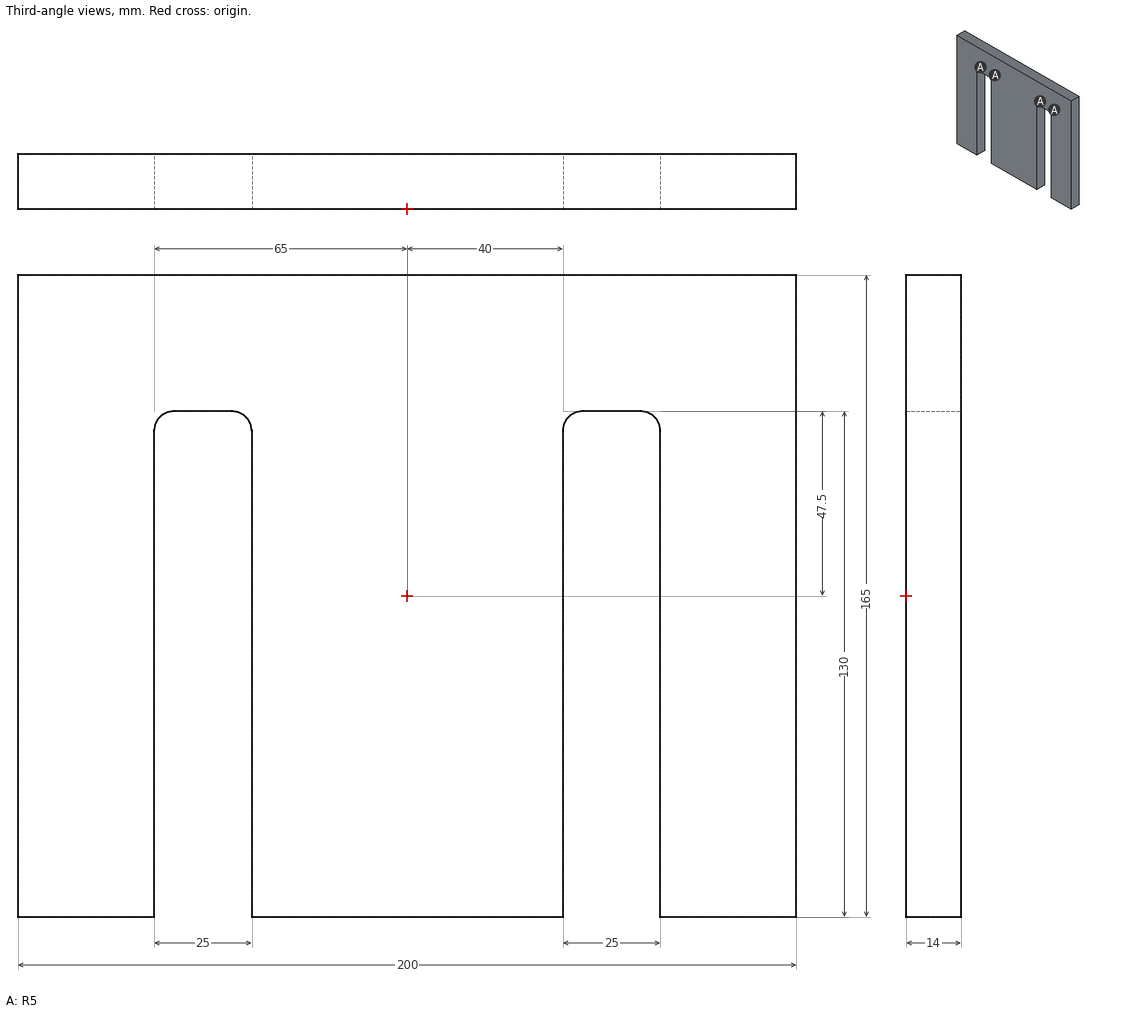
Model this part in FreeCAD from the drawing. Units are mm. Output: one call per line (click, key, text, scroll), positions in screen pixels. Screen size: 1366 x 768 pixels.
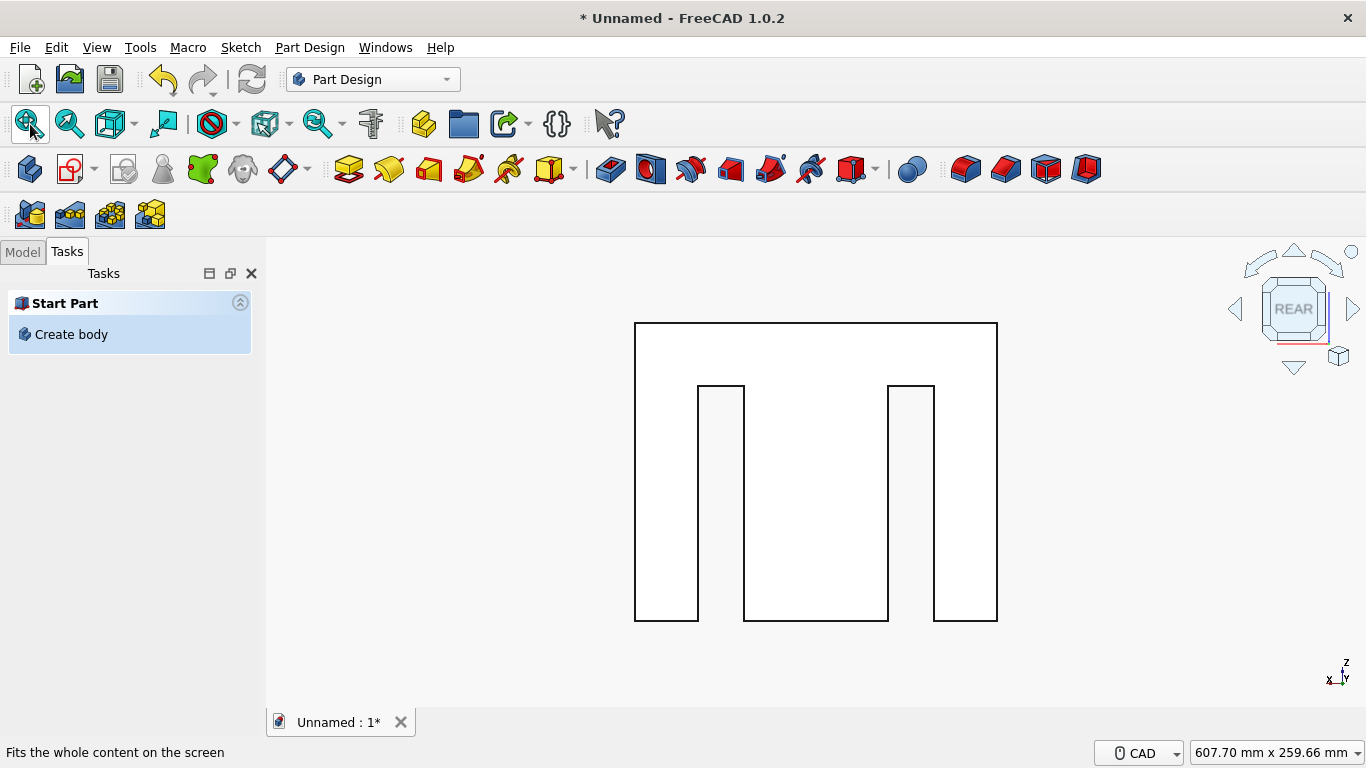
key(6)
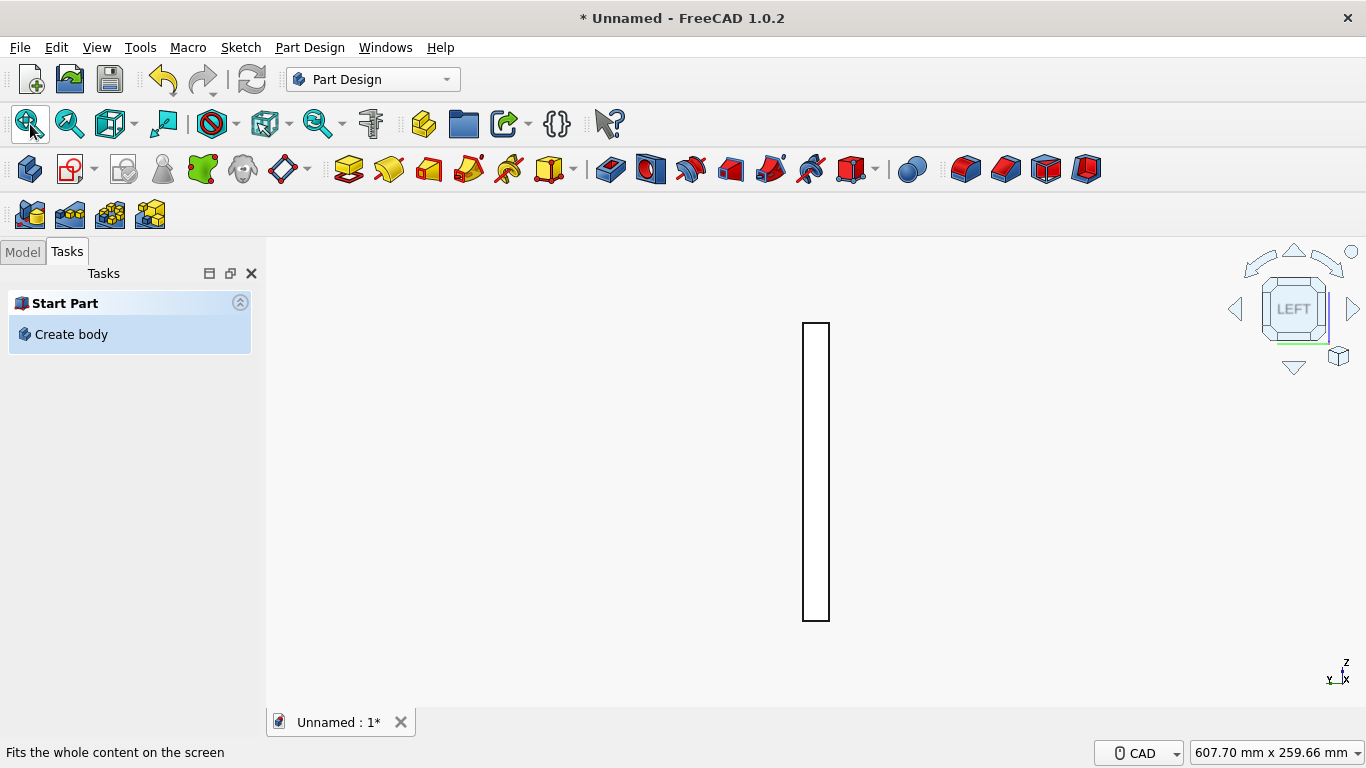
key(v)
key(3)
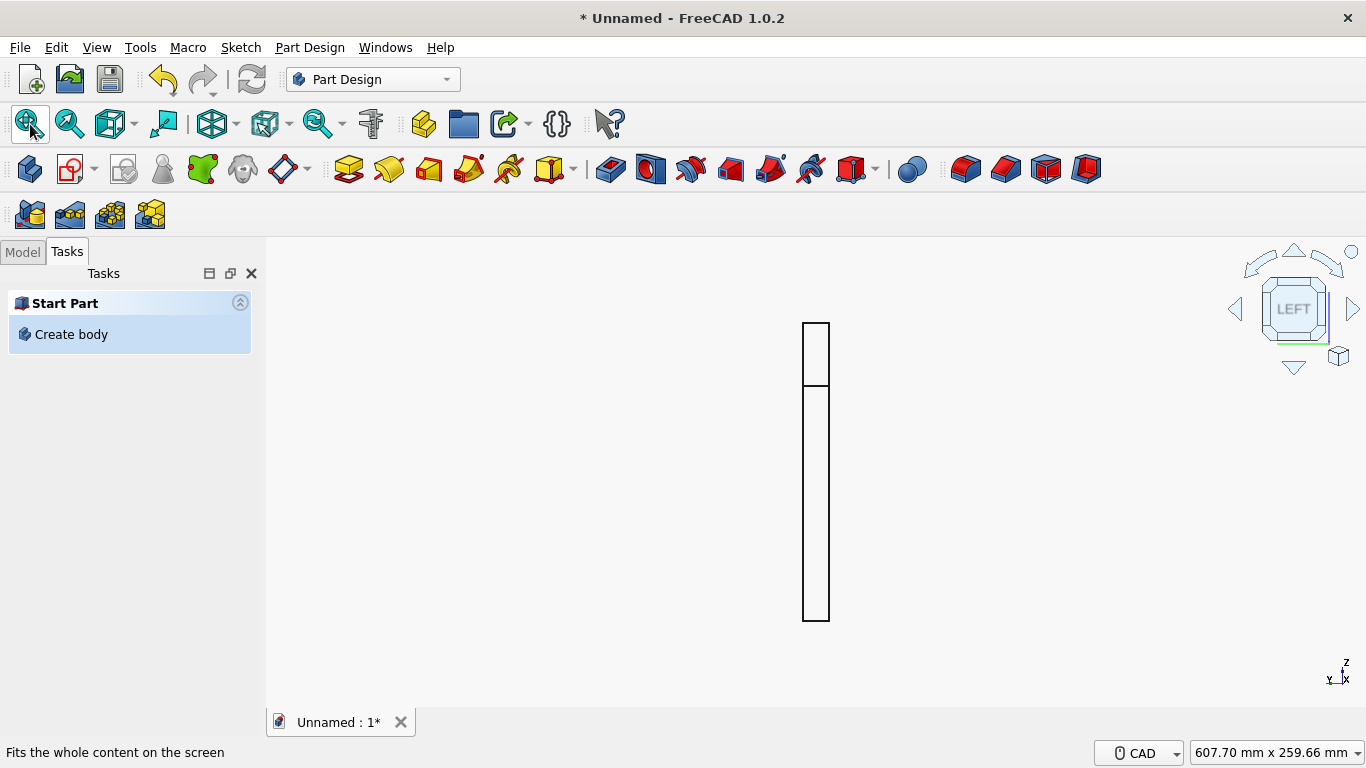
key(0)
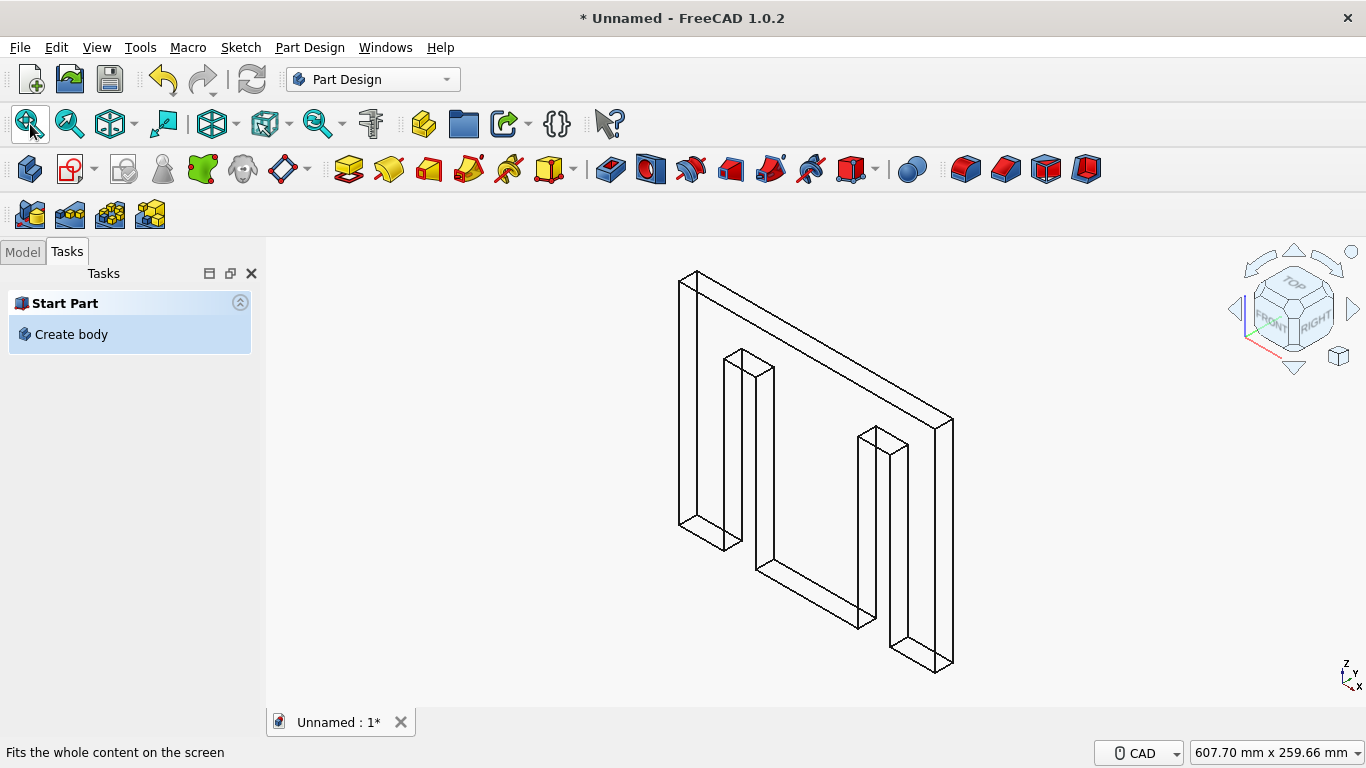
click(867, 430)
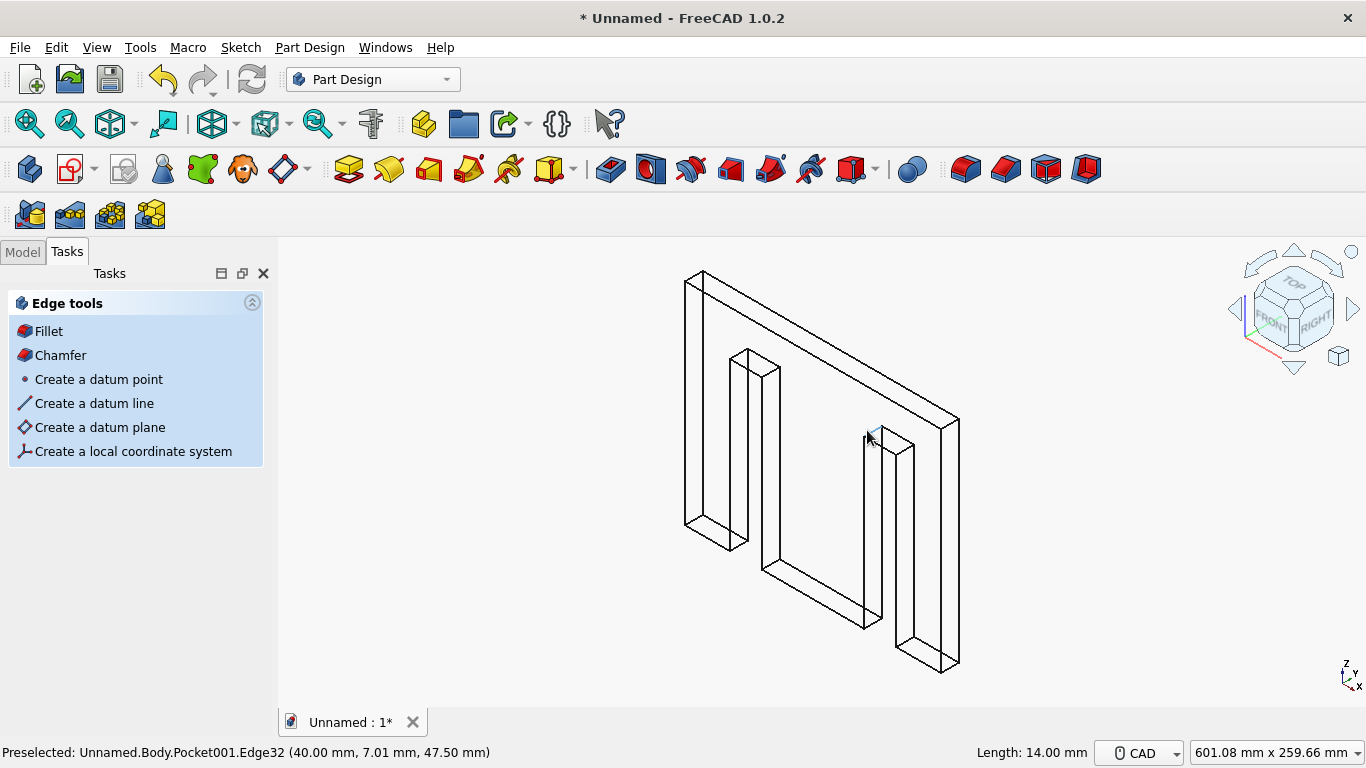
click(905, 449, ctrl)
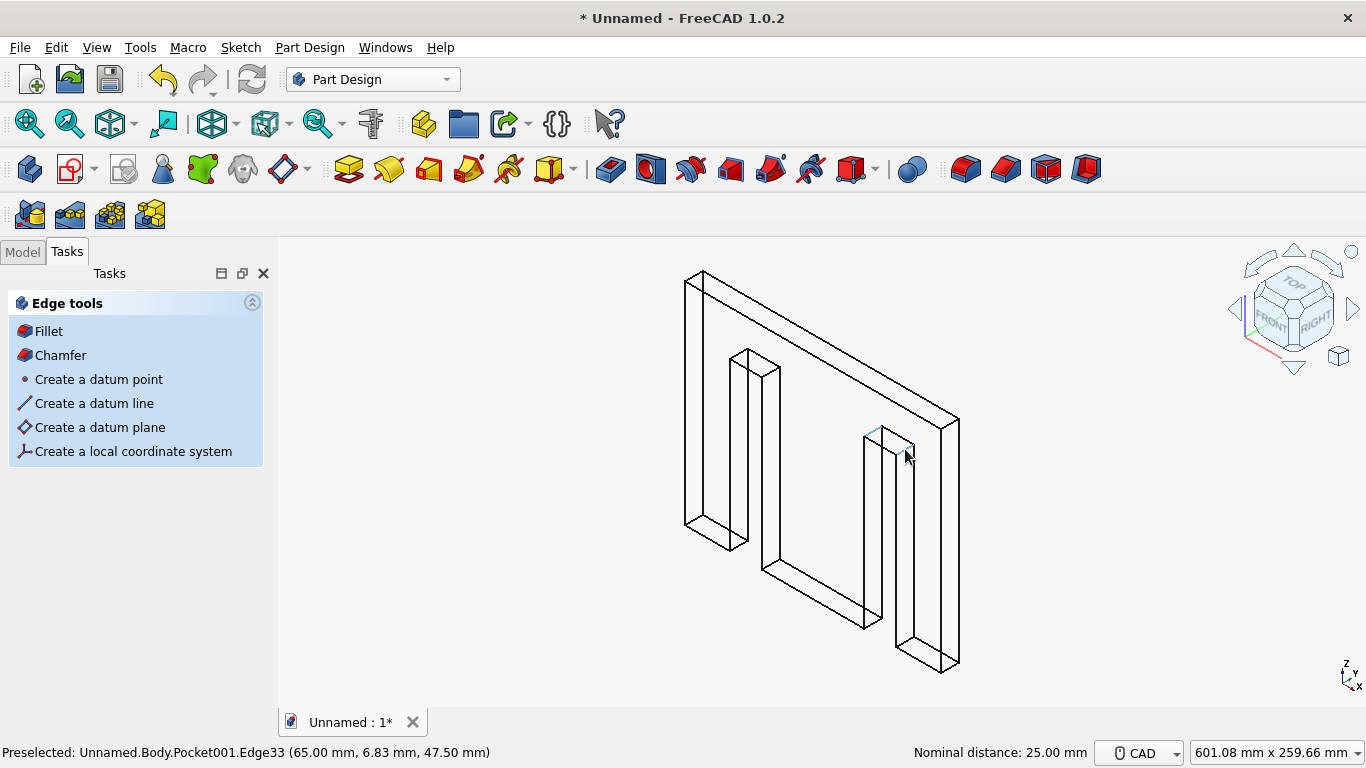
click(771, 371, ctrl)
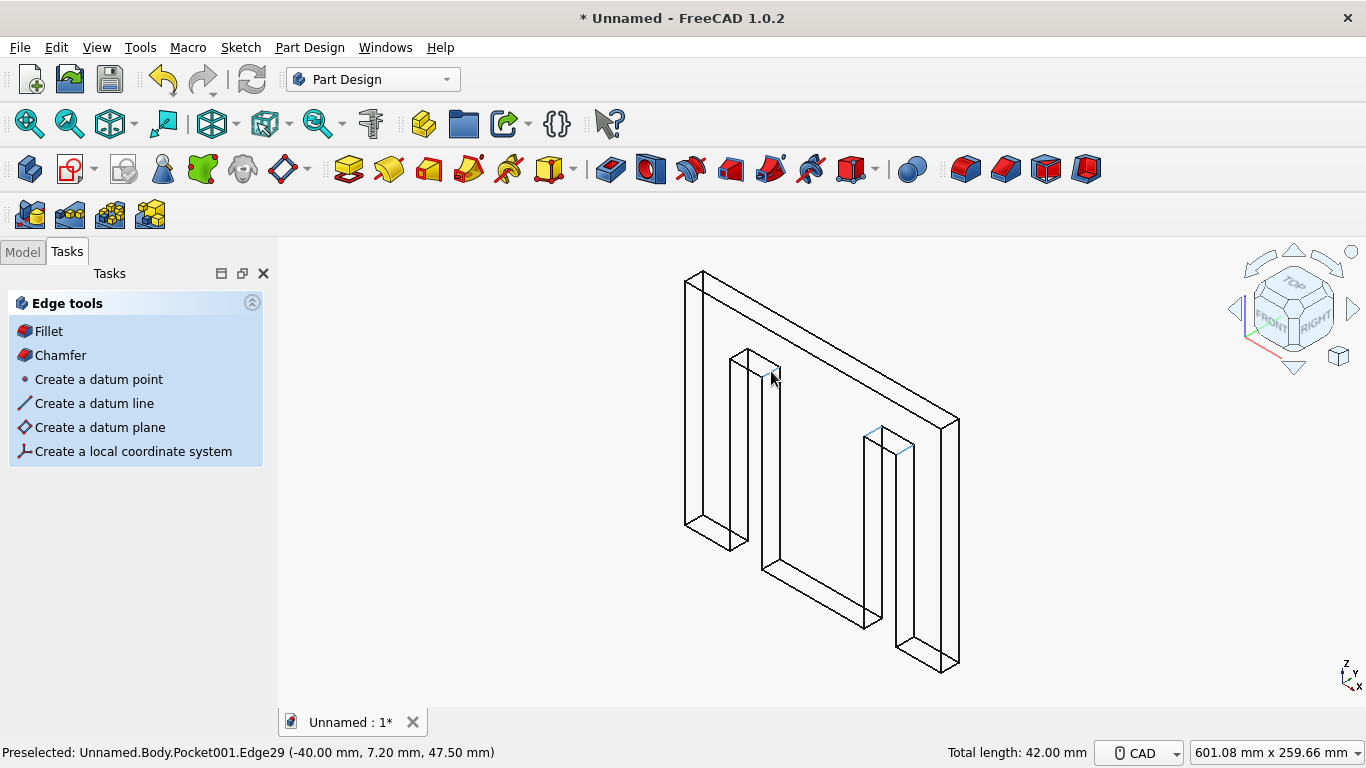
click(739, 353, ctrl)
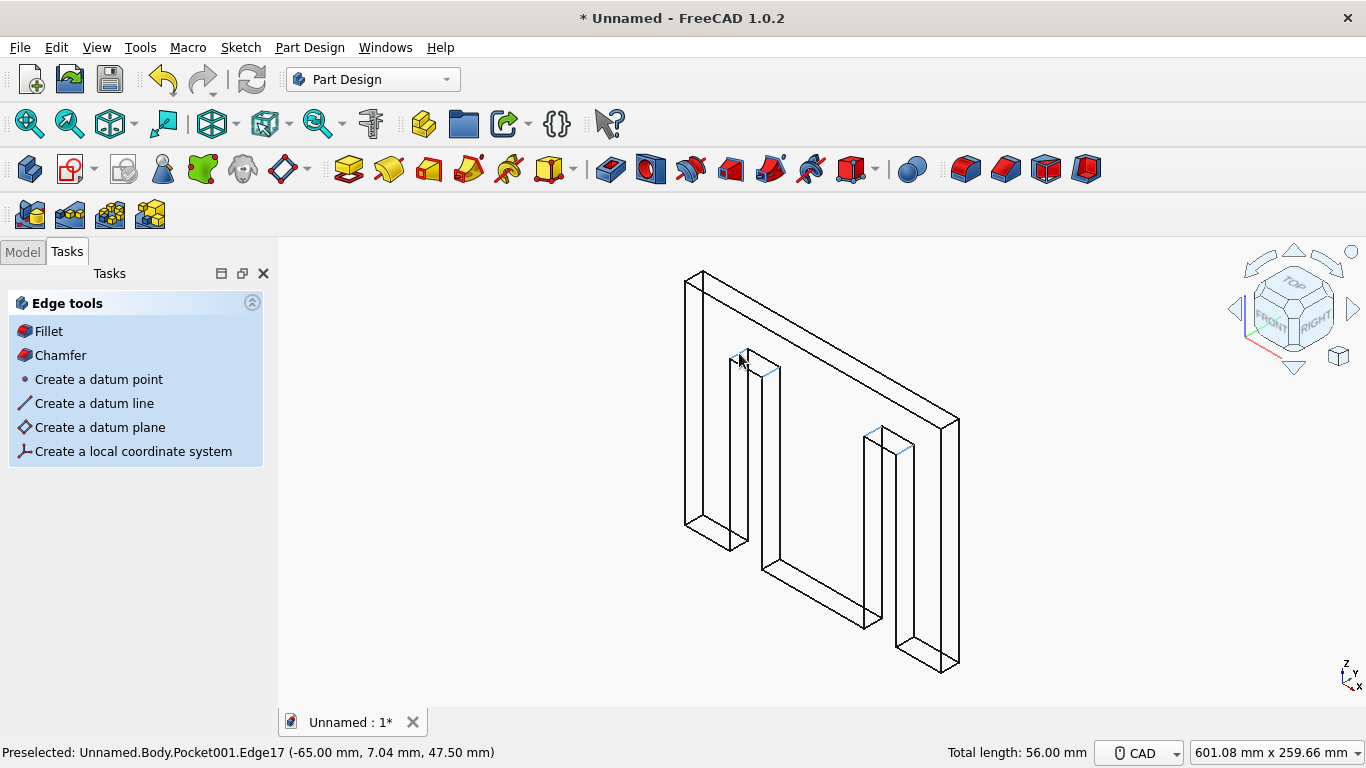
key(v)
key(1)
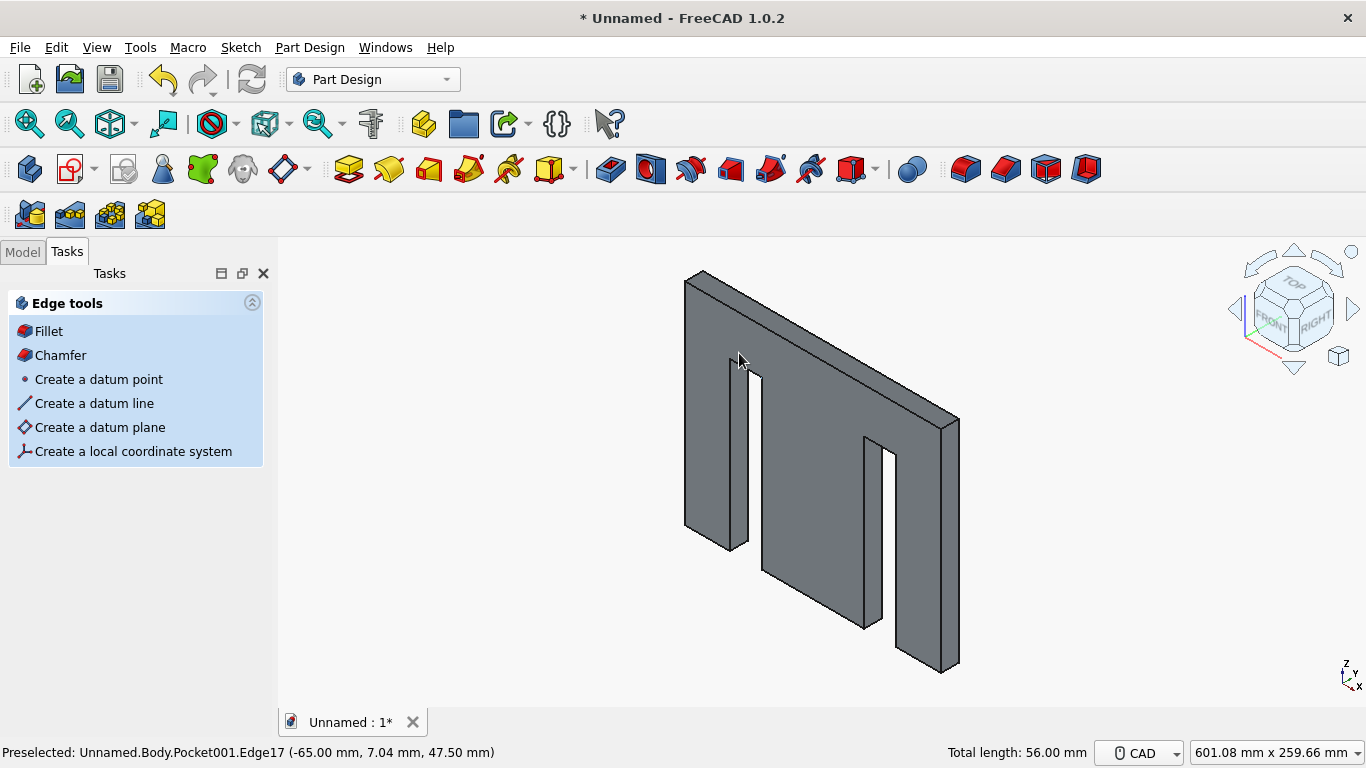
click(966, 170)